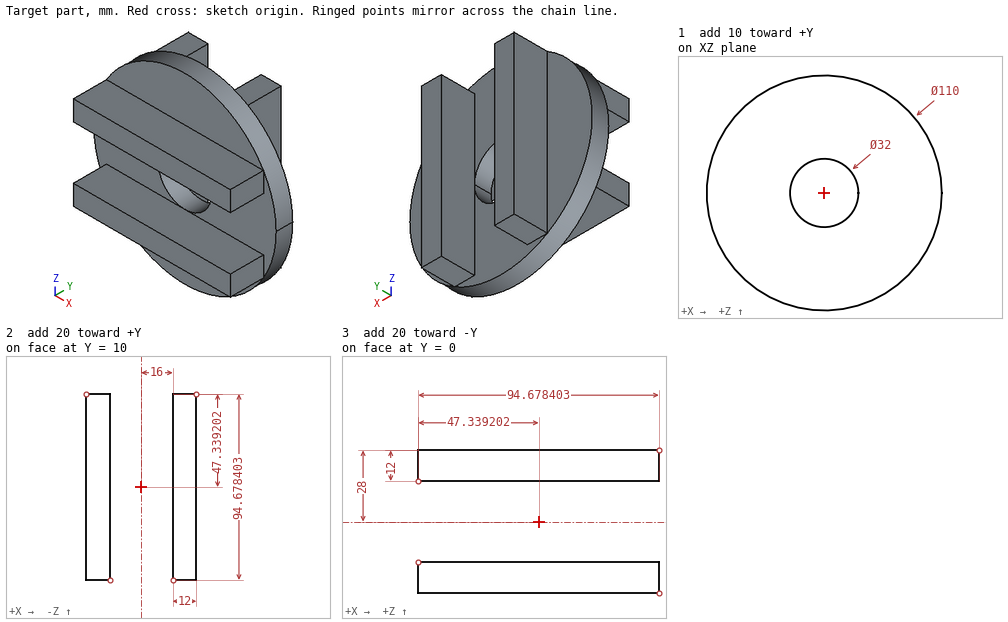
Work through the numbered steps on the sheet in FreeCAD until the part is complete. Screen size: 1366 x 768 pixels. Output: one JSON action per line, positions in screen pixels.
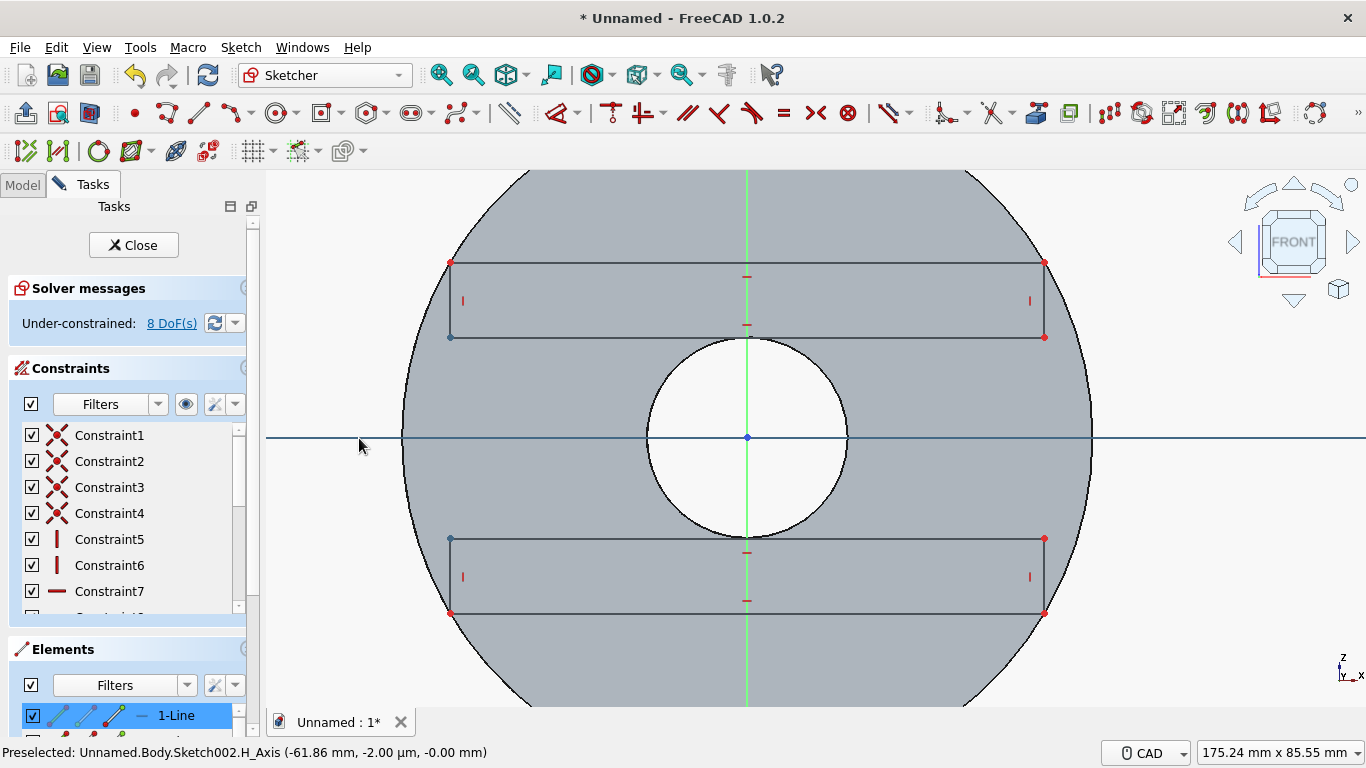
{"action": "left_click", "coordinate": [816, 114]}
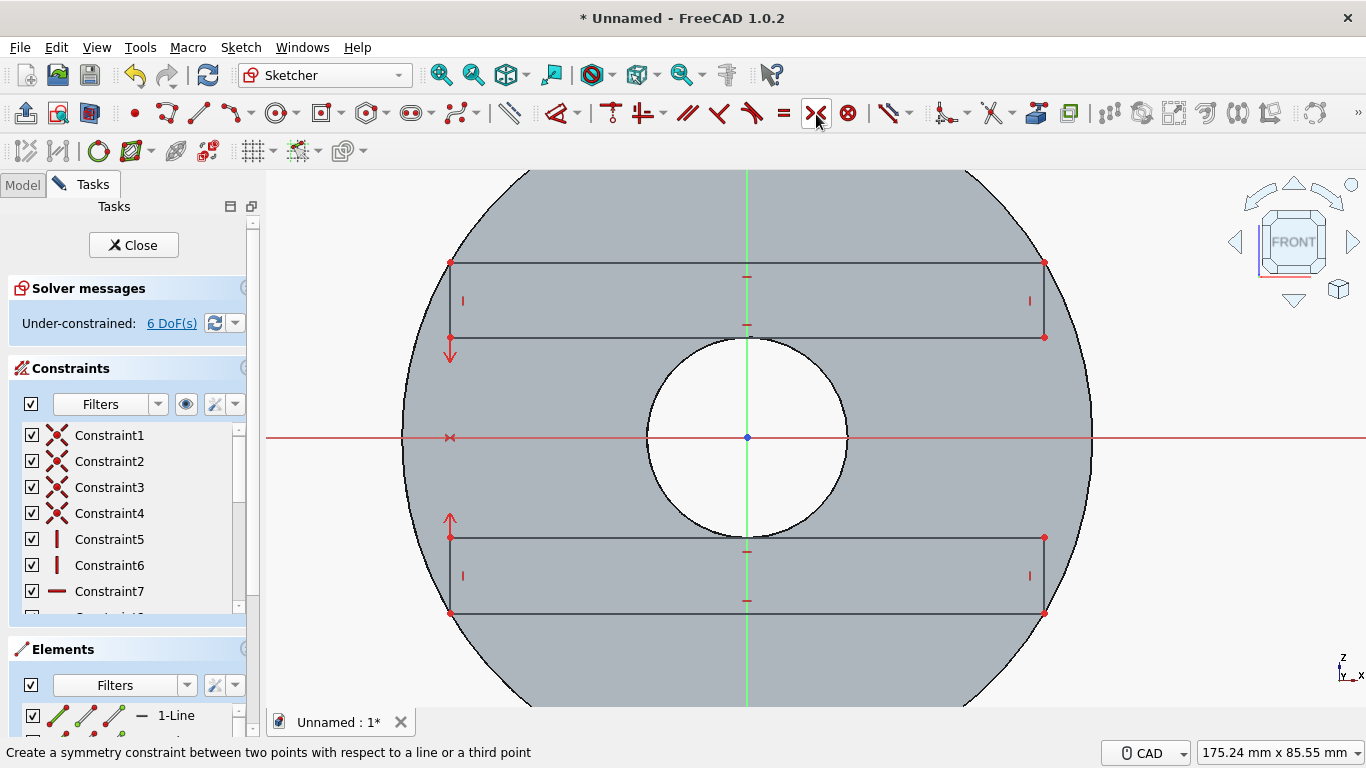
{"action": "left_click", "coordinate": [1044, 263]}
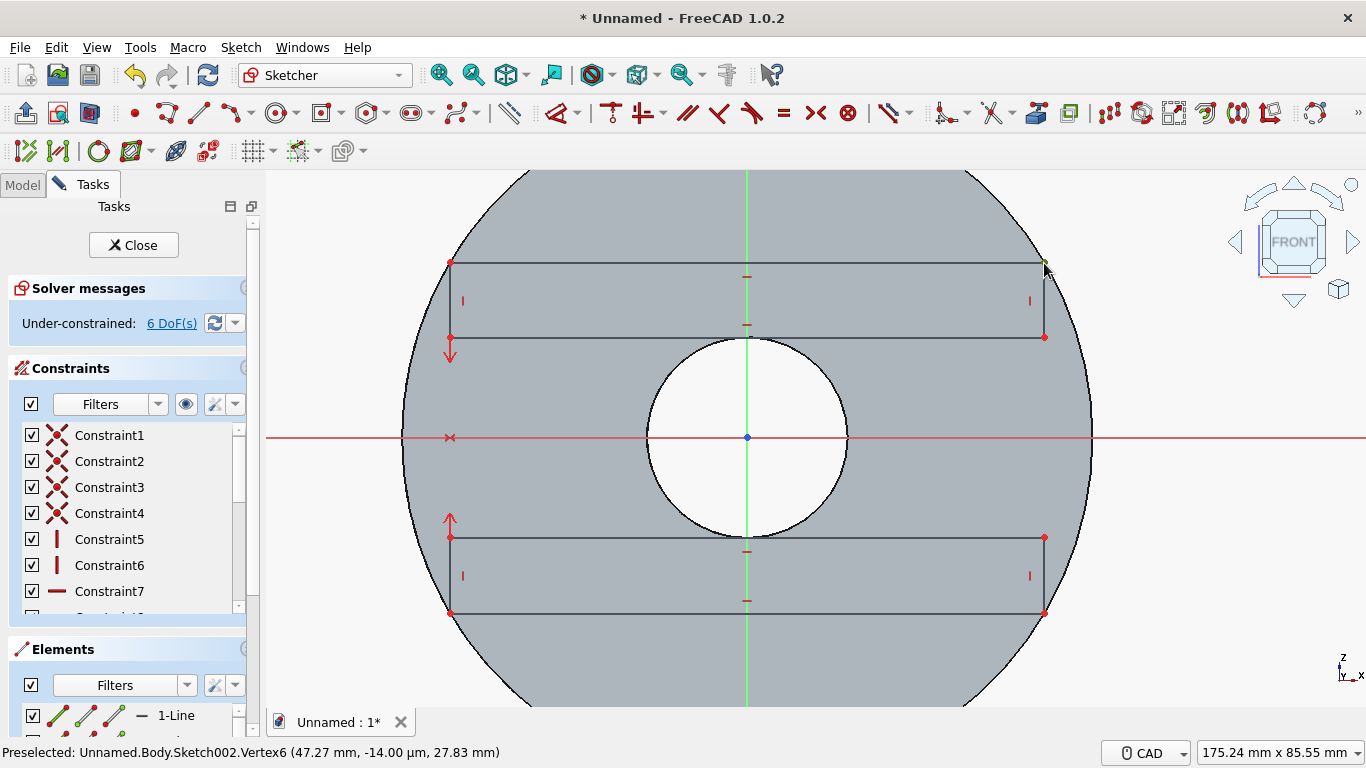
{"action": "left_click", "coordinate": [1044, 614]}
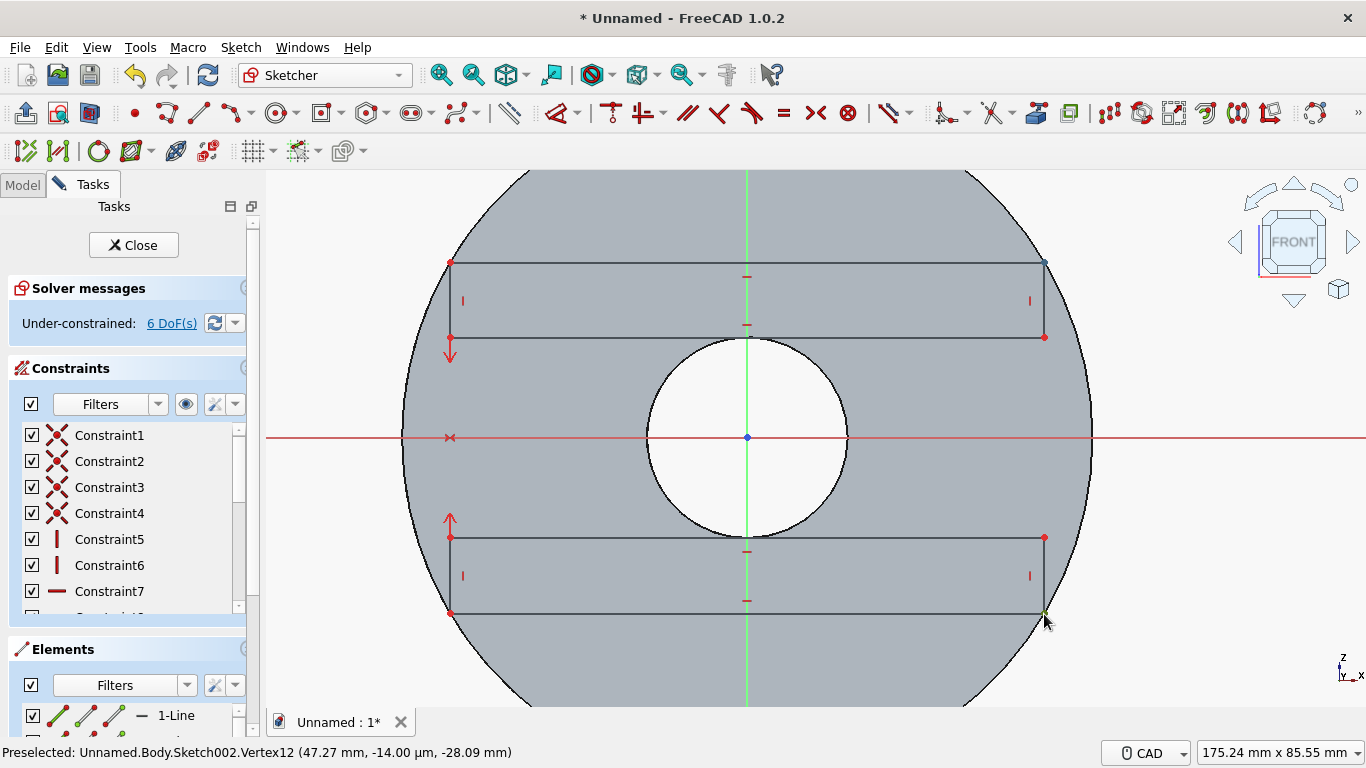
{"action": "left_click", "coordinate": [359, 438]}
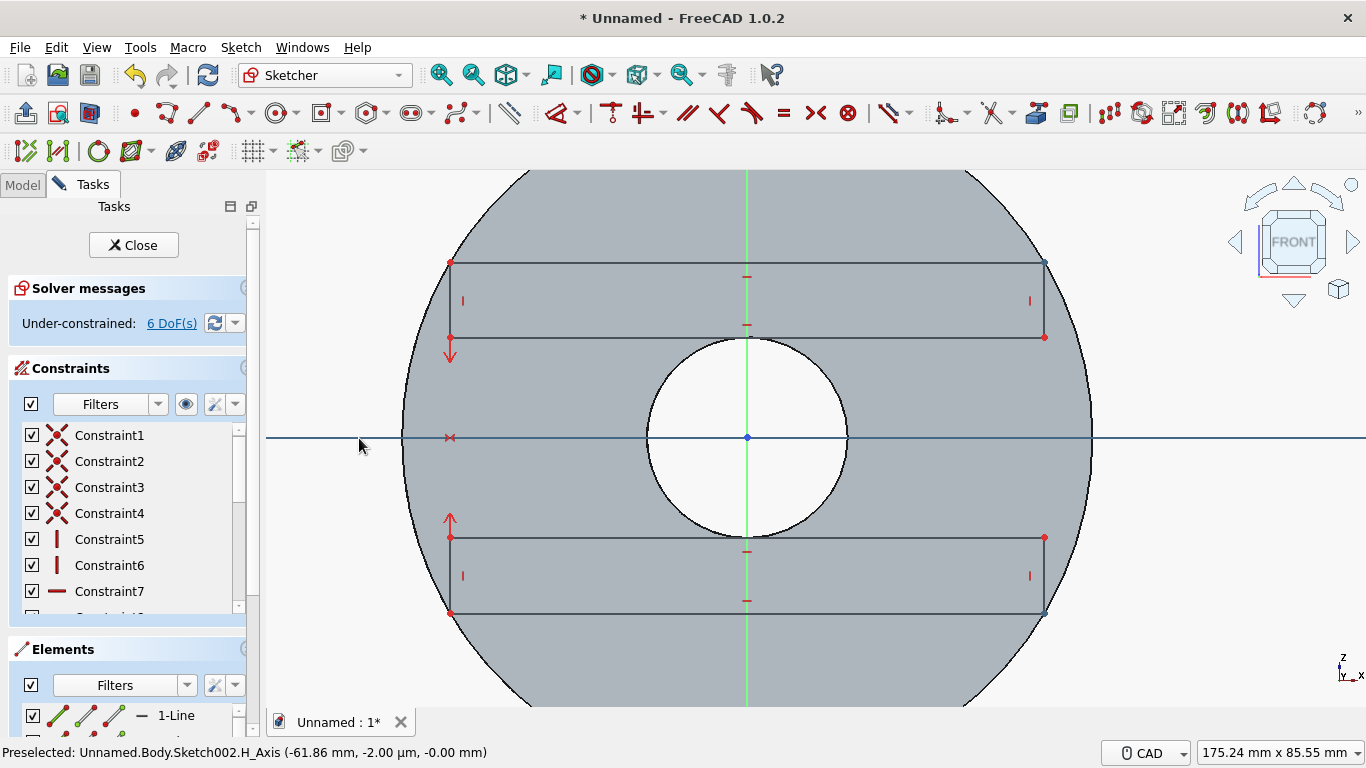
{"action": "left_click", "coordinate": [816, 114]}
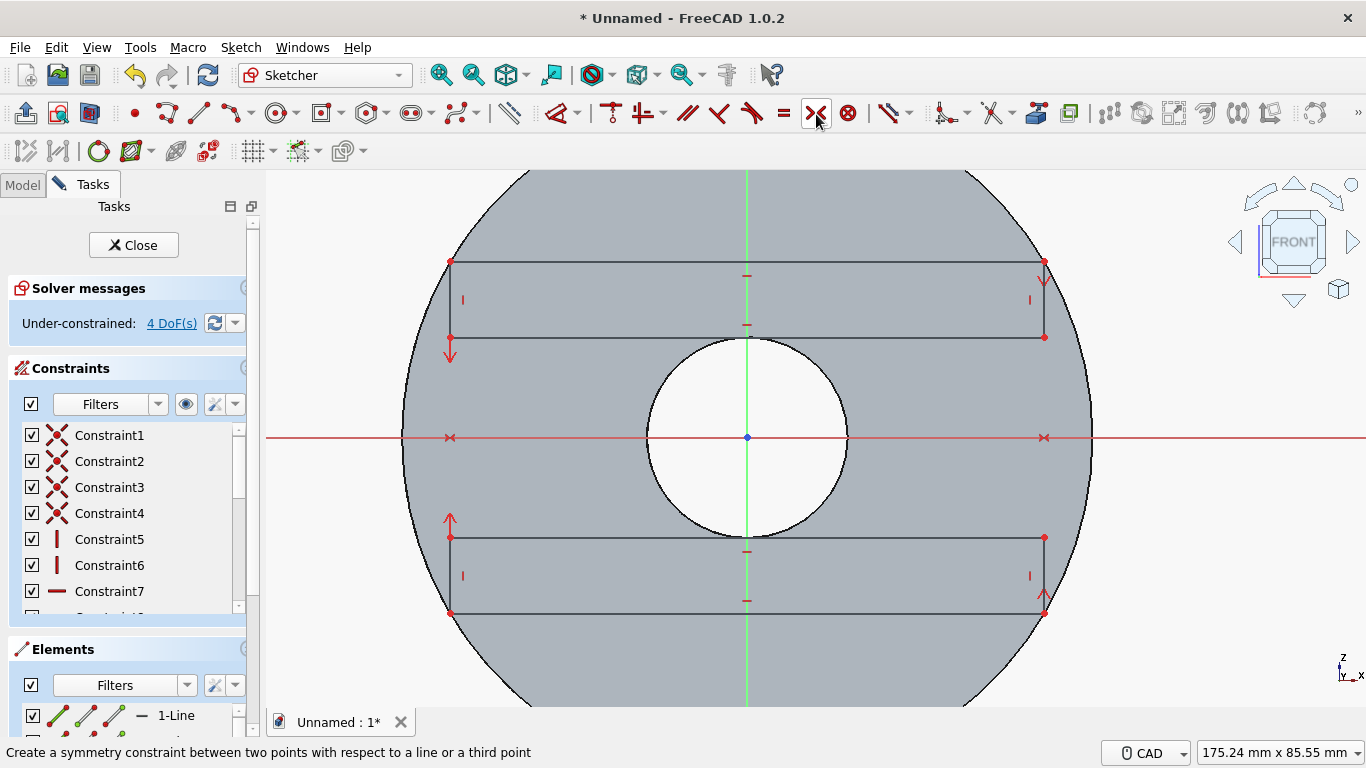
{"action": "left_click", "coordinate": [450, 285]}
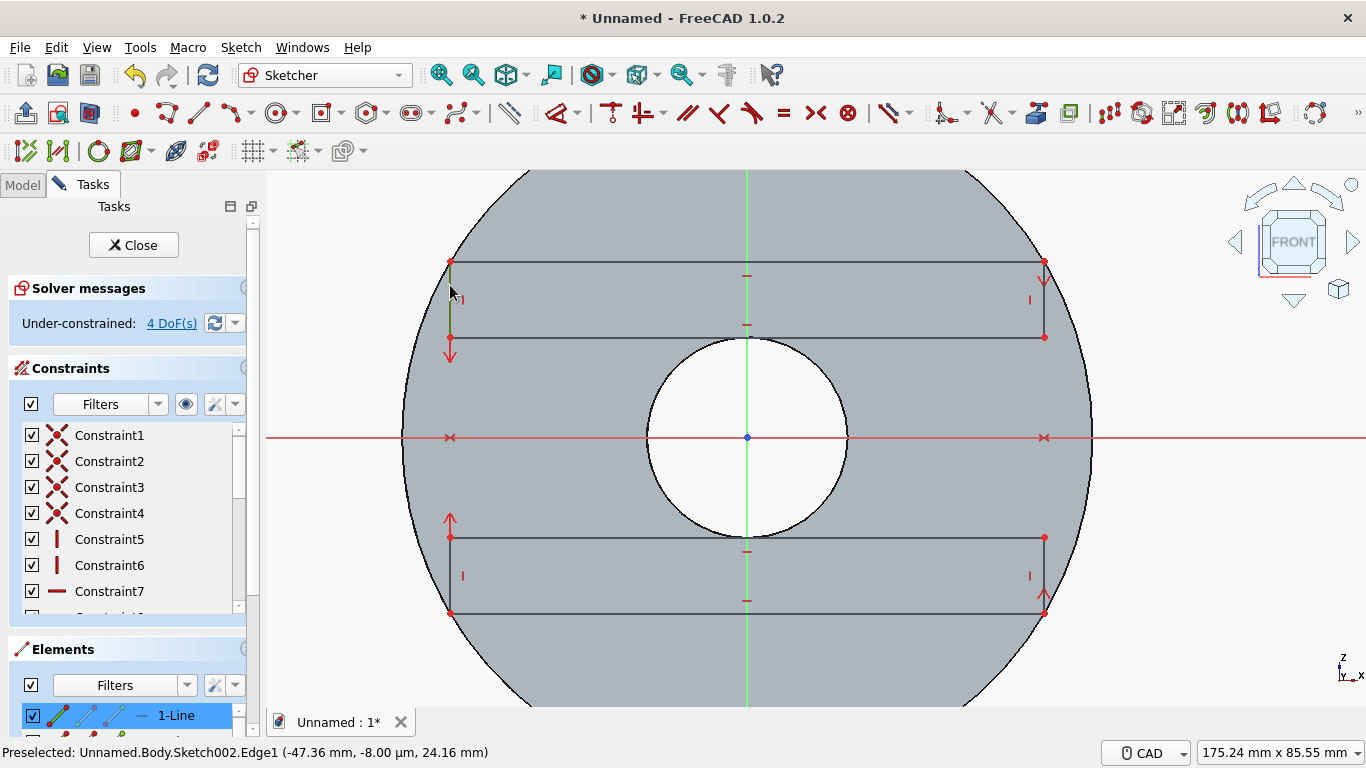
{"action": "key", "text": "i"}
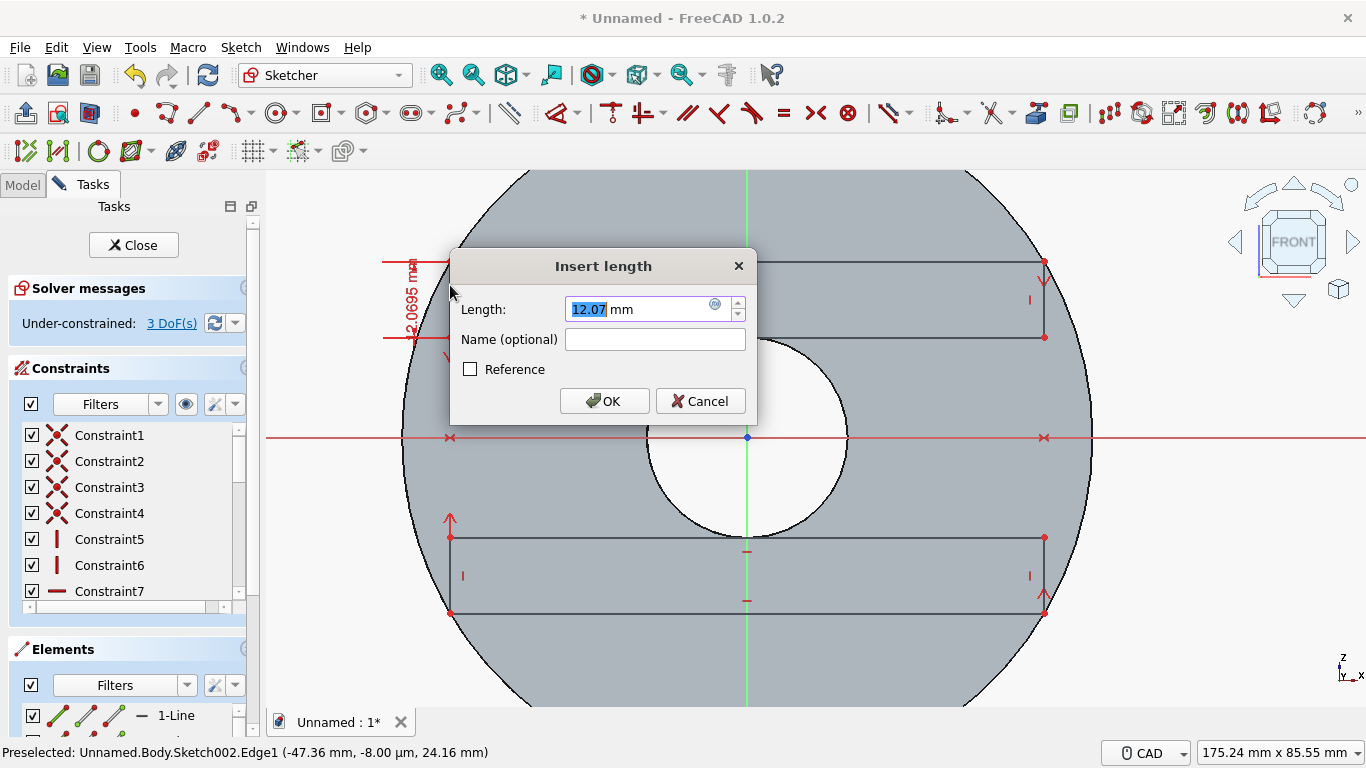
{"action": "type", "text": "12"}
{"action": "key", "text": "Return"}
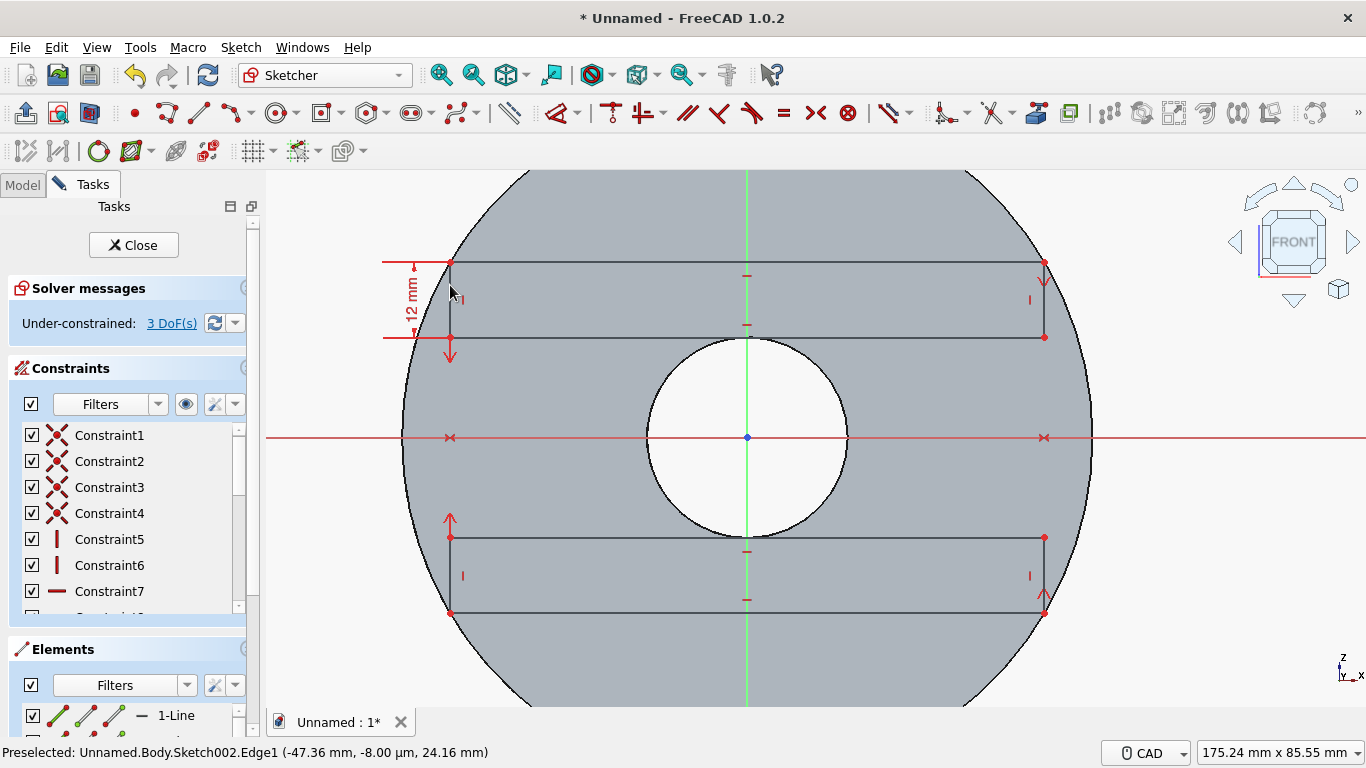
{"action": "left_click", "coordinate": [450, 262]}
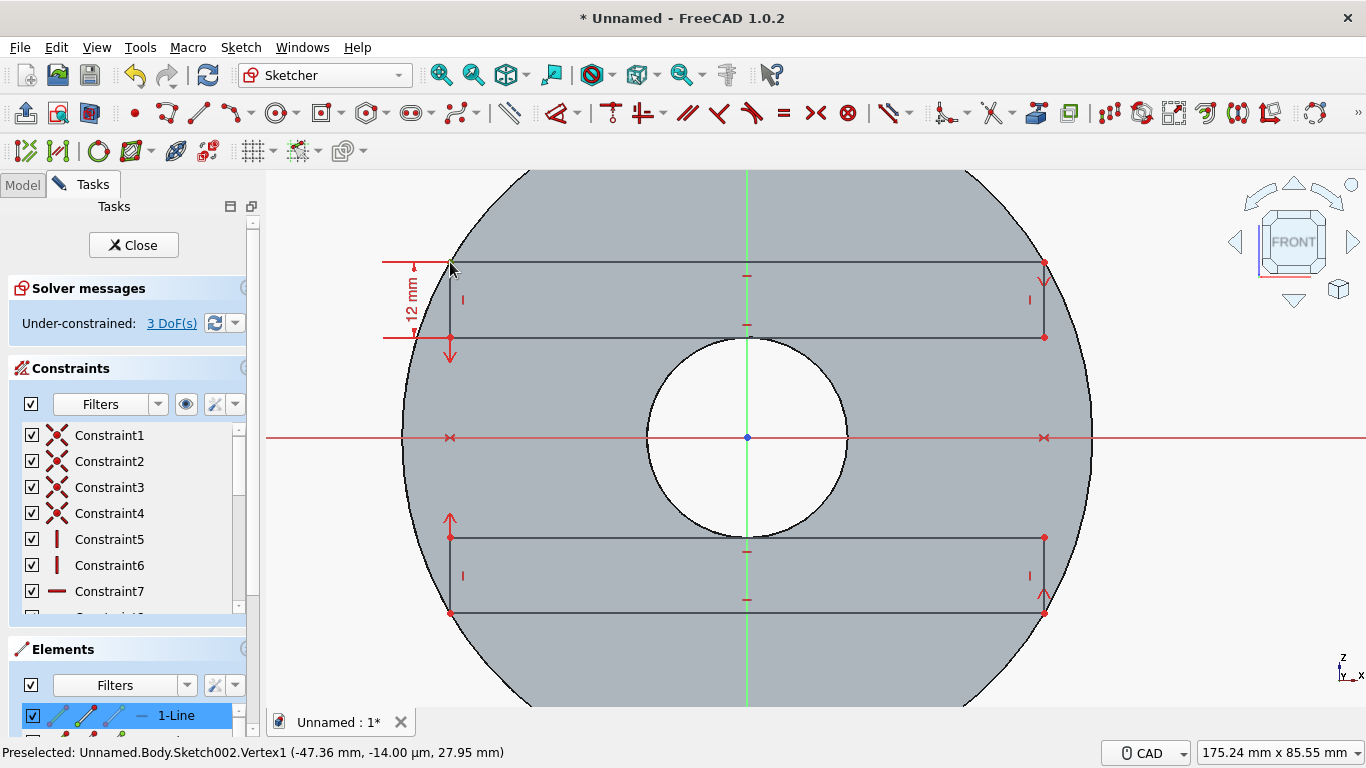
{"action": "key", "text": "i"}